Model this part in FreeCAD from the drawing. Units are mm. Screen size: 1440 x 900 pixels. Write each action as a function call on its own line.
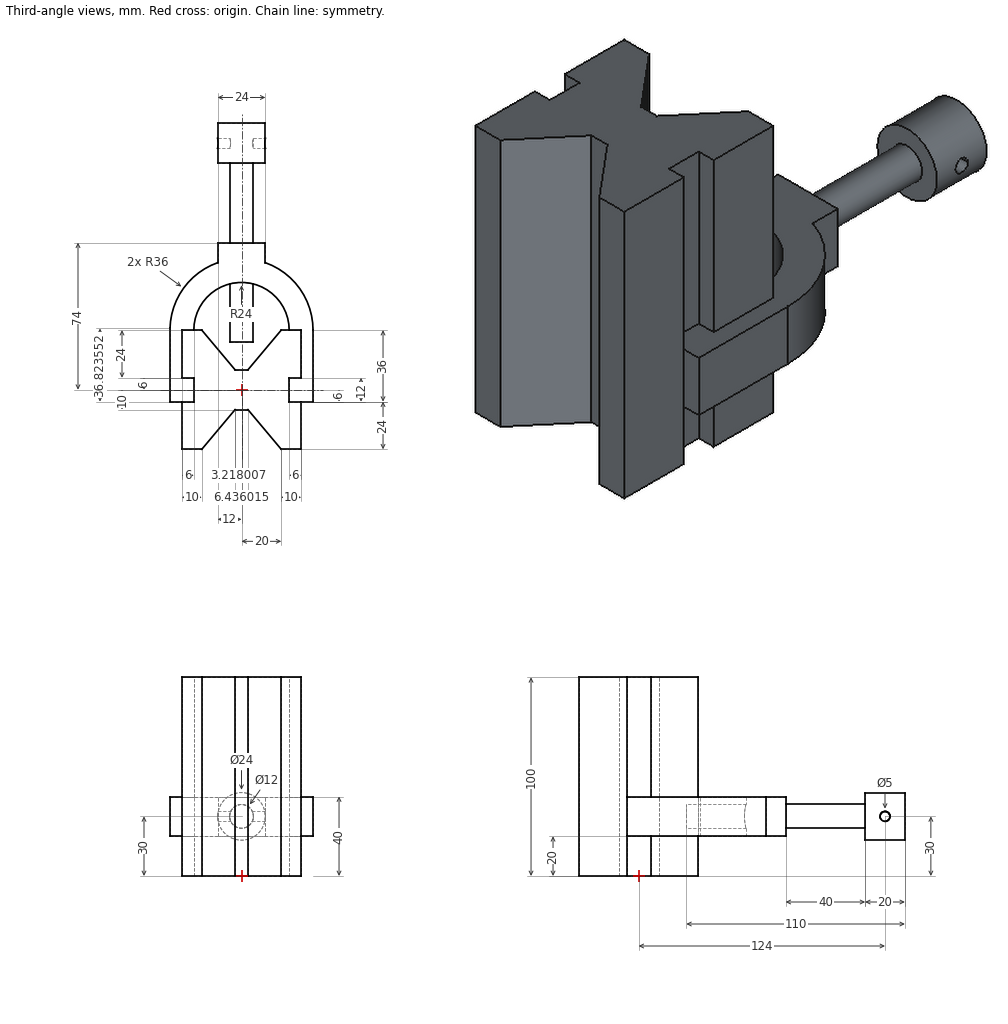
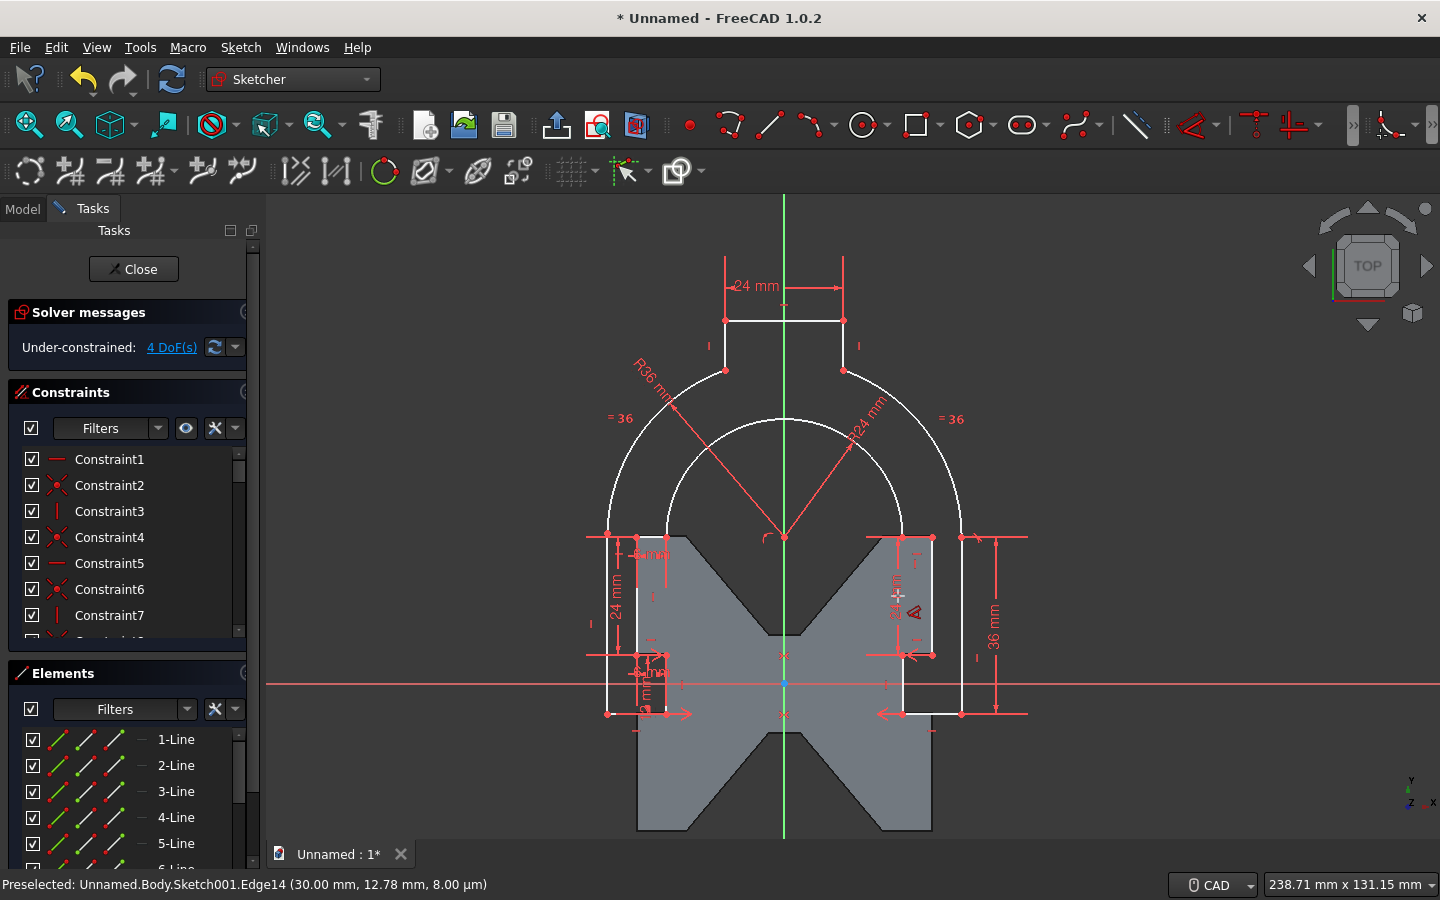
scroll(637, 655, up, 2)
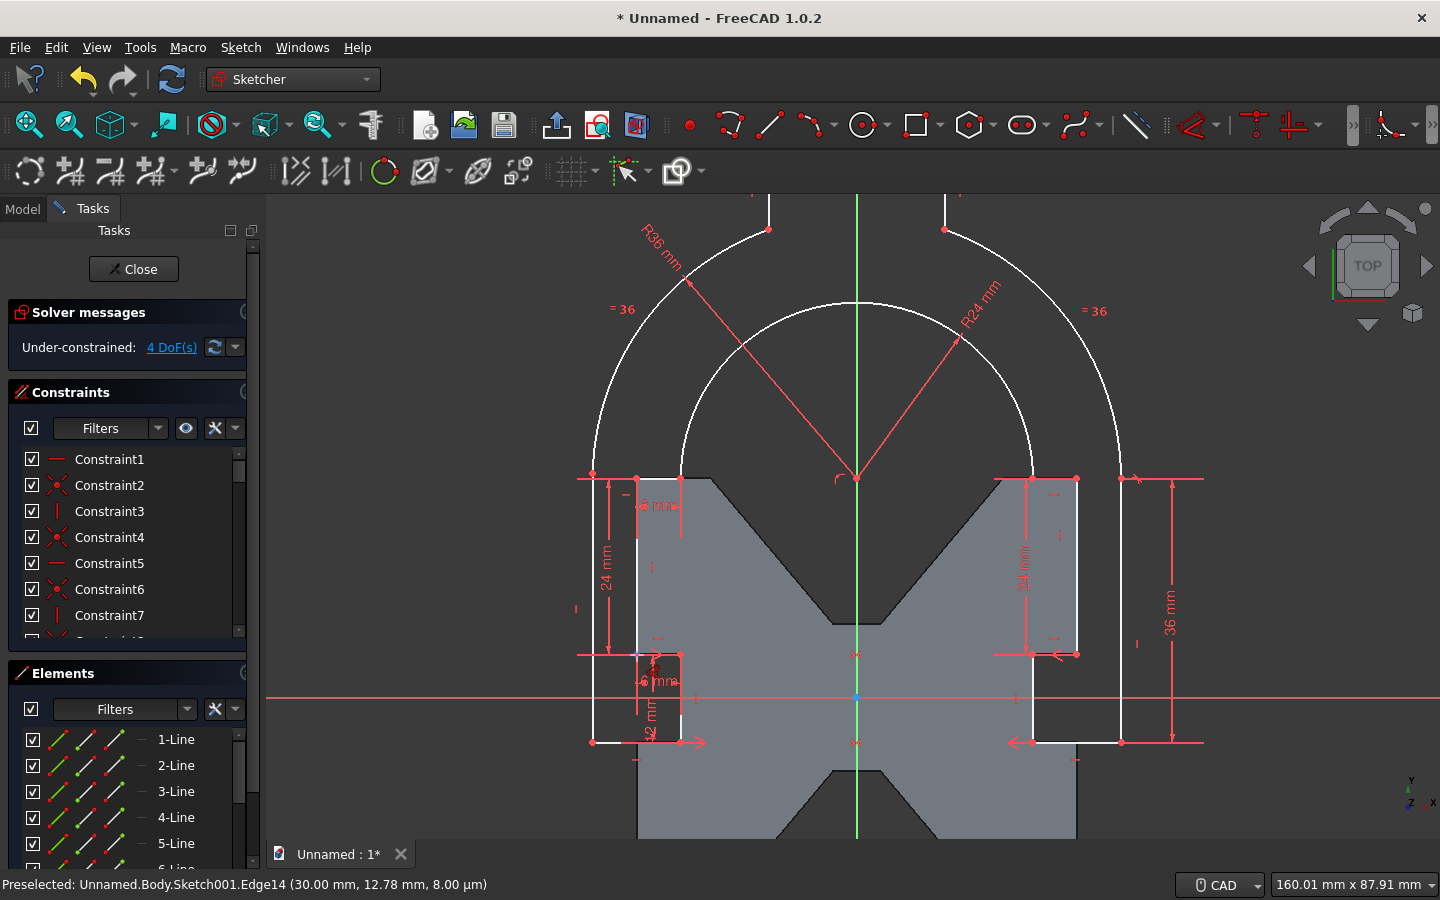
click(637, 655)
click(891, 676)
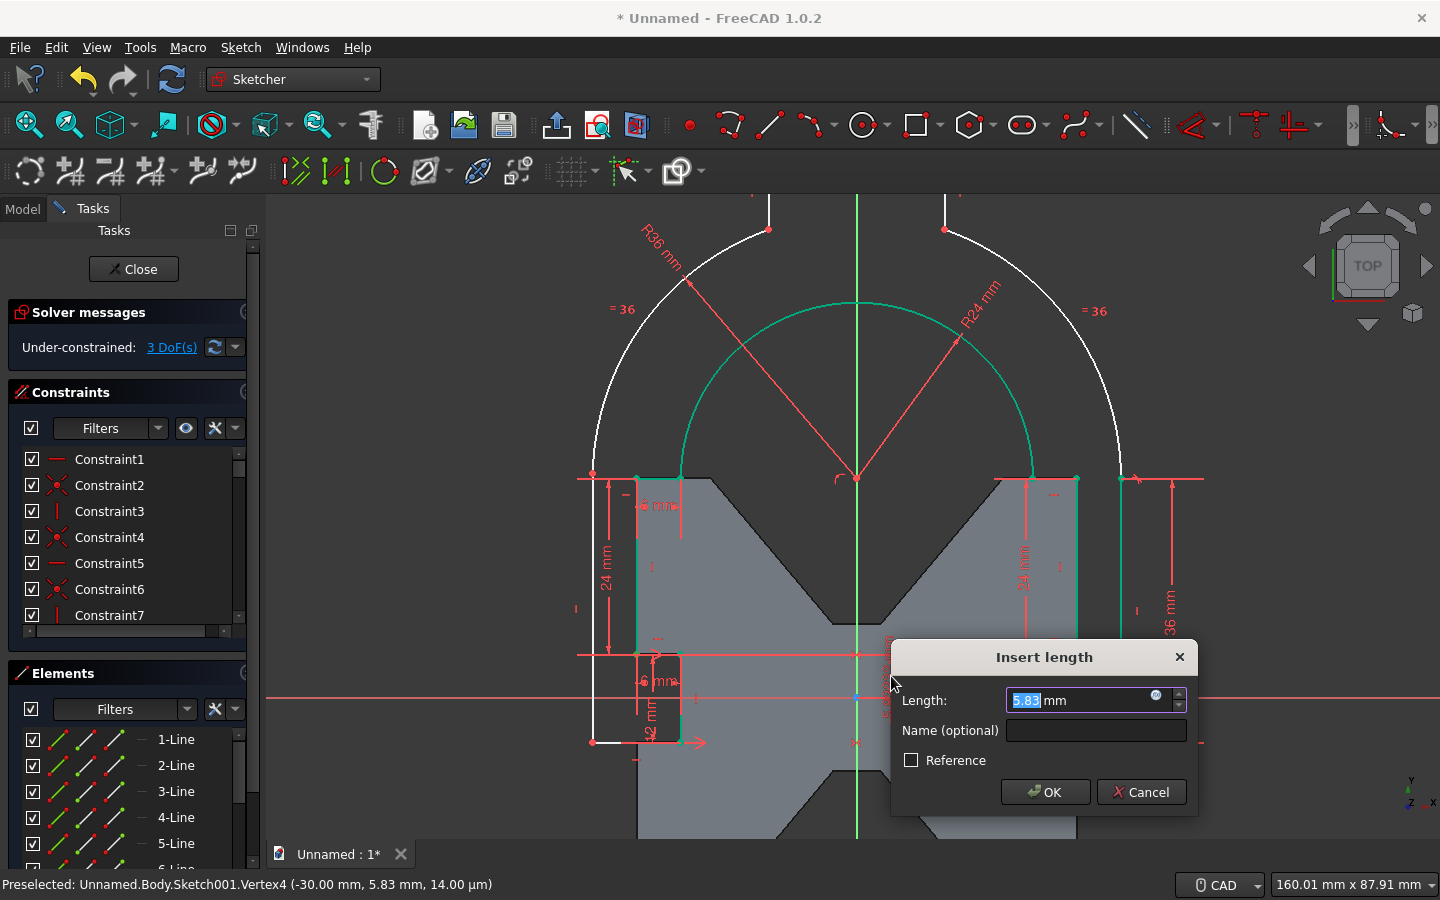
text(6)
key(Return)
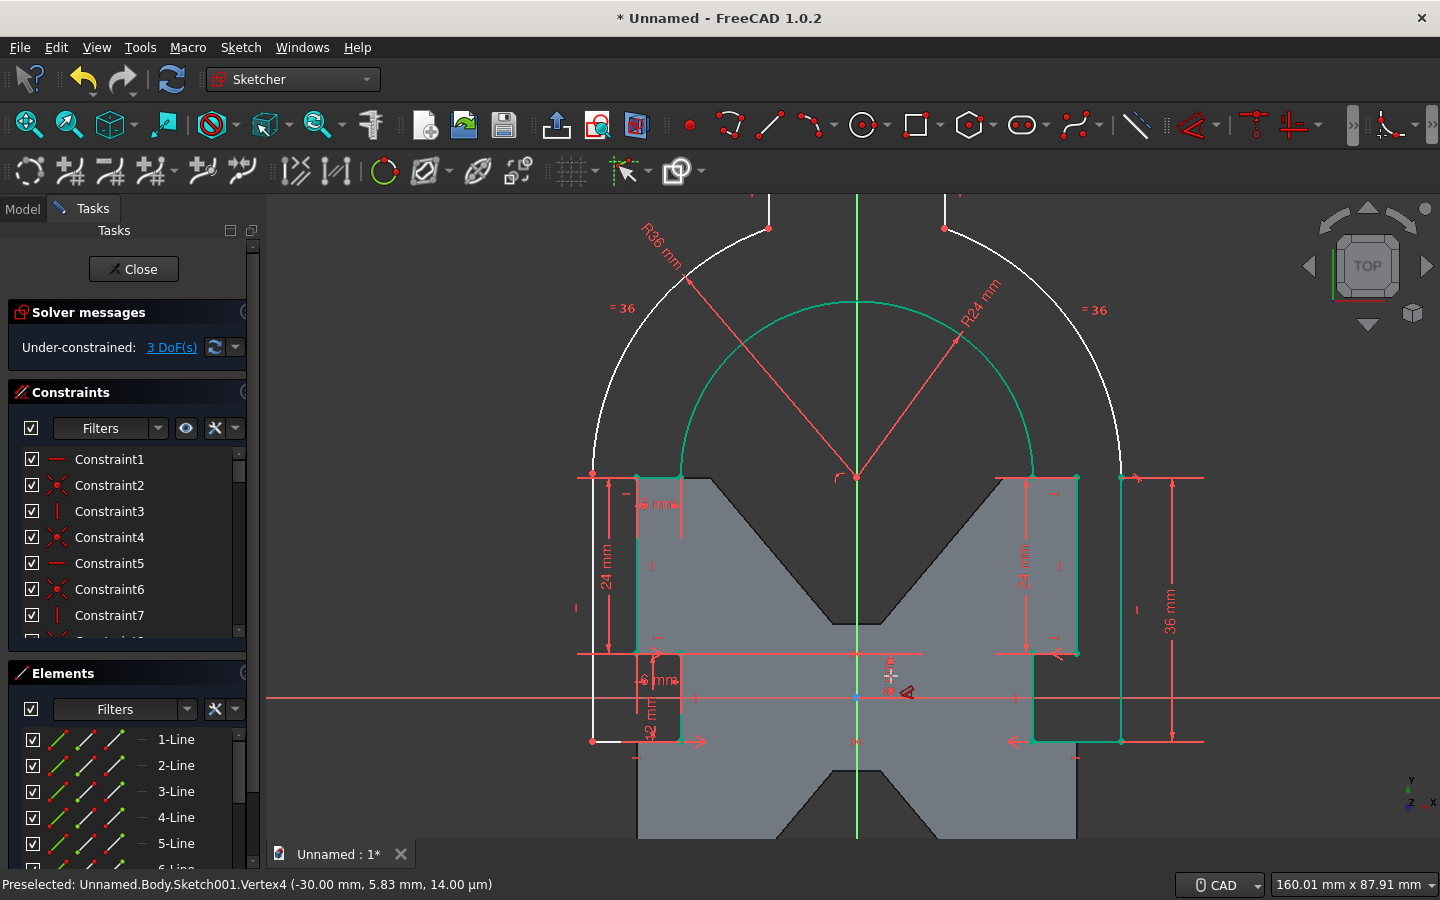
click(769, 229)
click(813, 732)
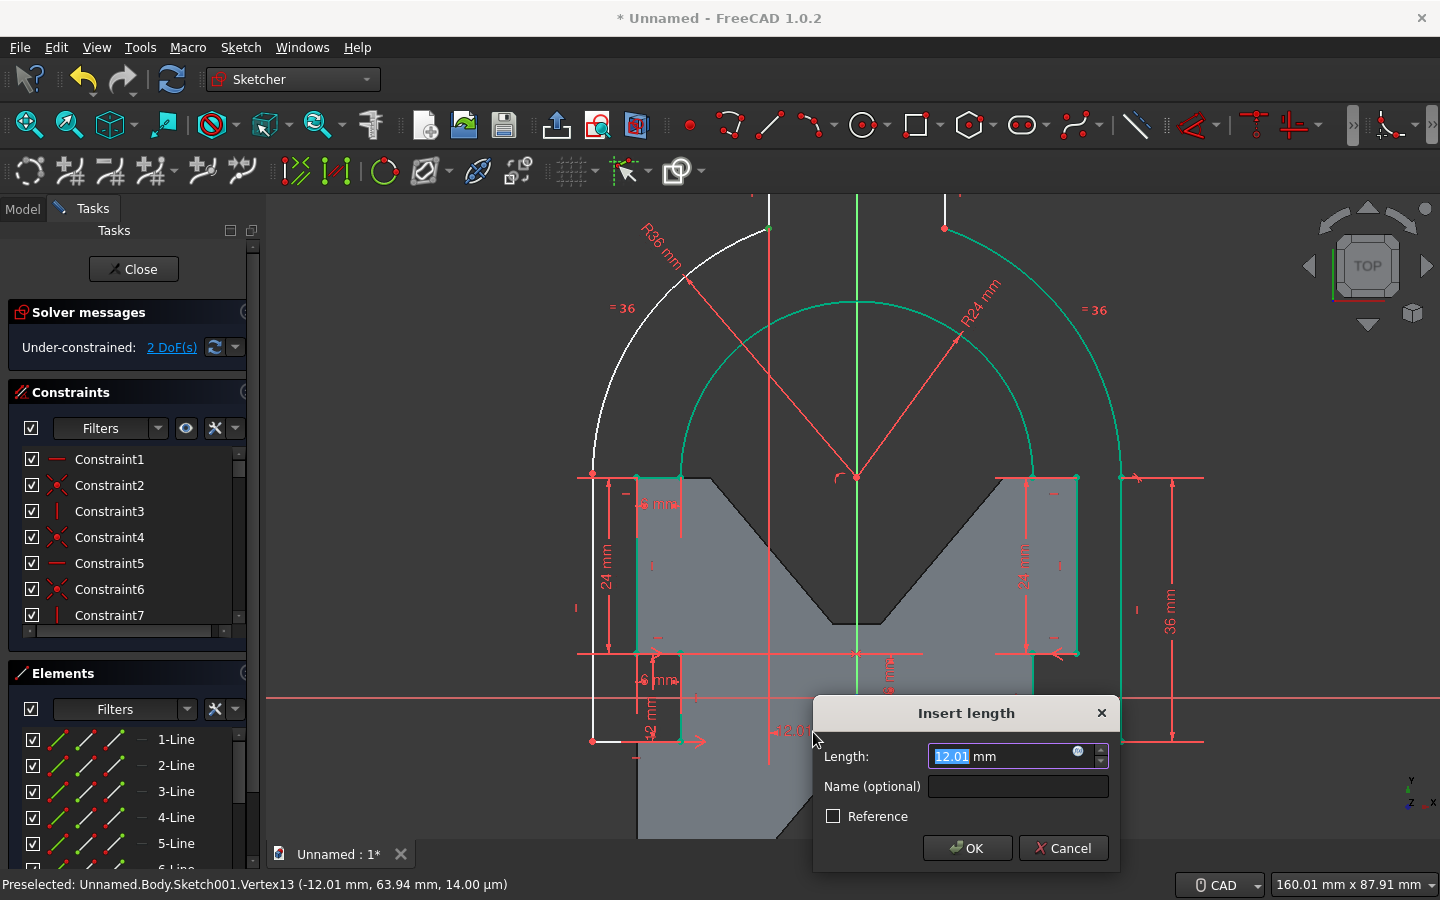
text(12)
key(Return)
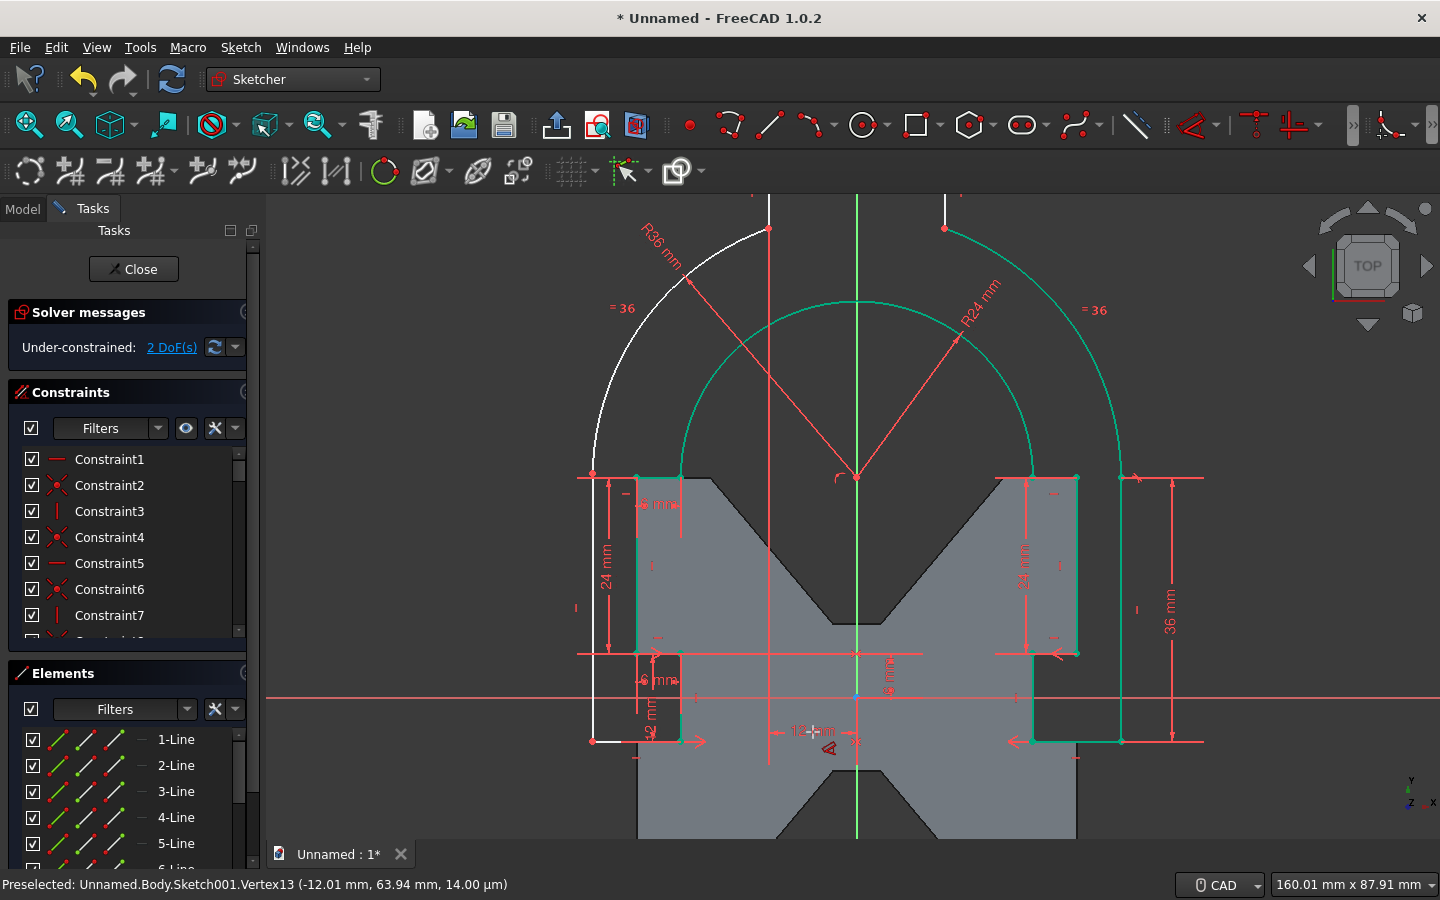
scroll(637, 655, down, 2)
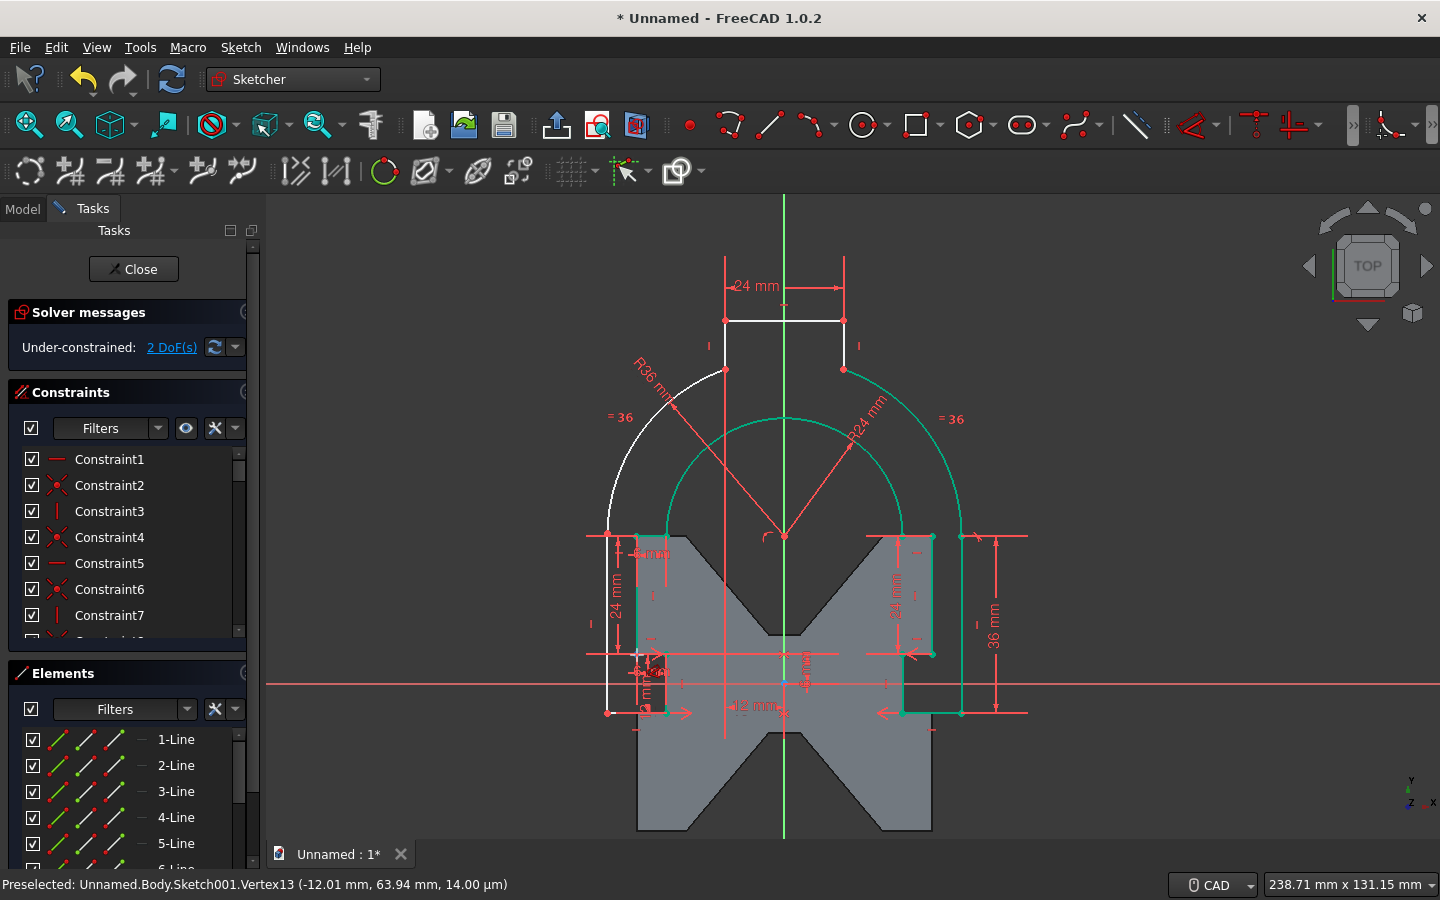
click(725, 321)
click(691, 502)